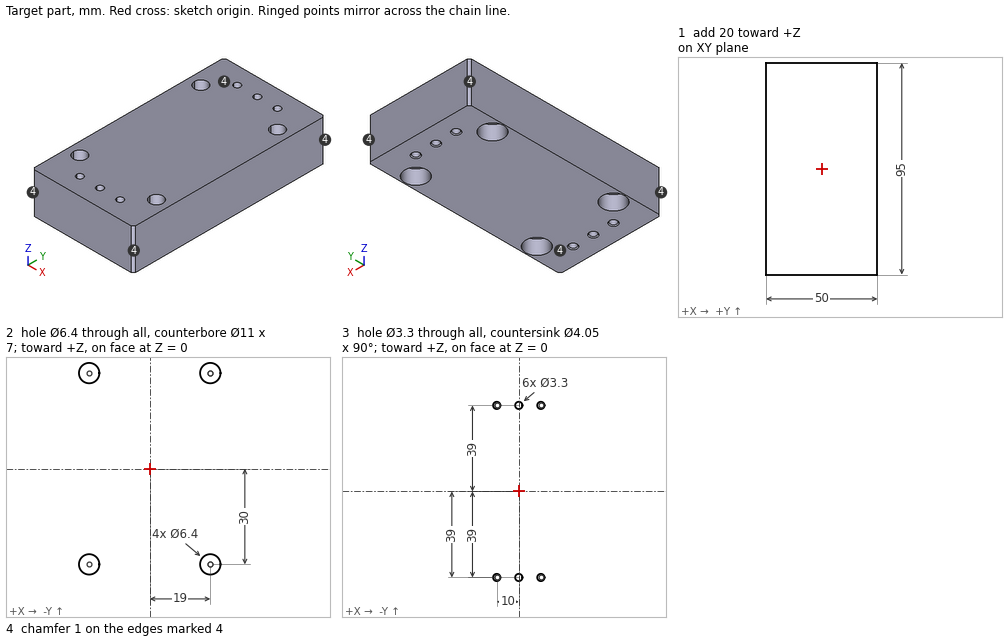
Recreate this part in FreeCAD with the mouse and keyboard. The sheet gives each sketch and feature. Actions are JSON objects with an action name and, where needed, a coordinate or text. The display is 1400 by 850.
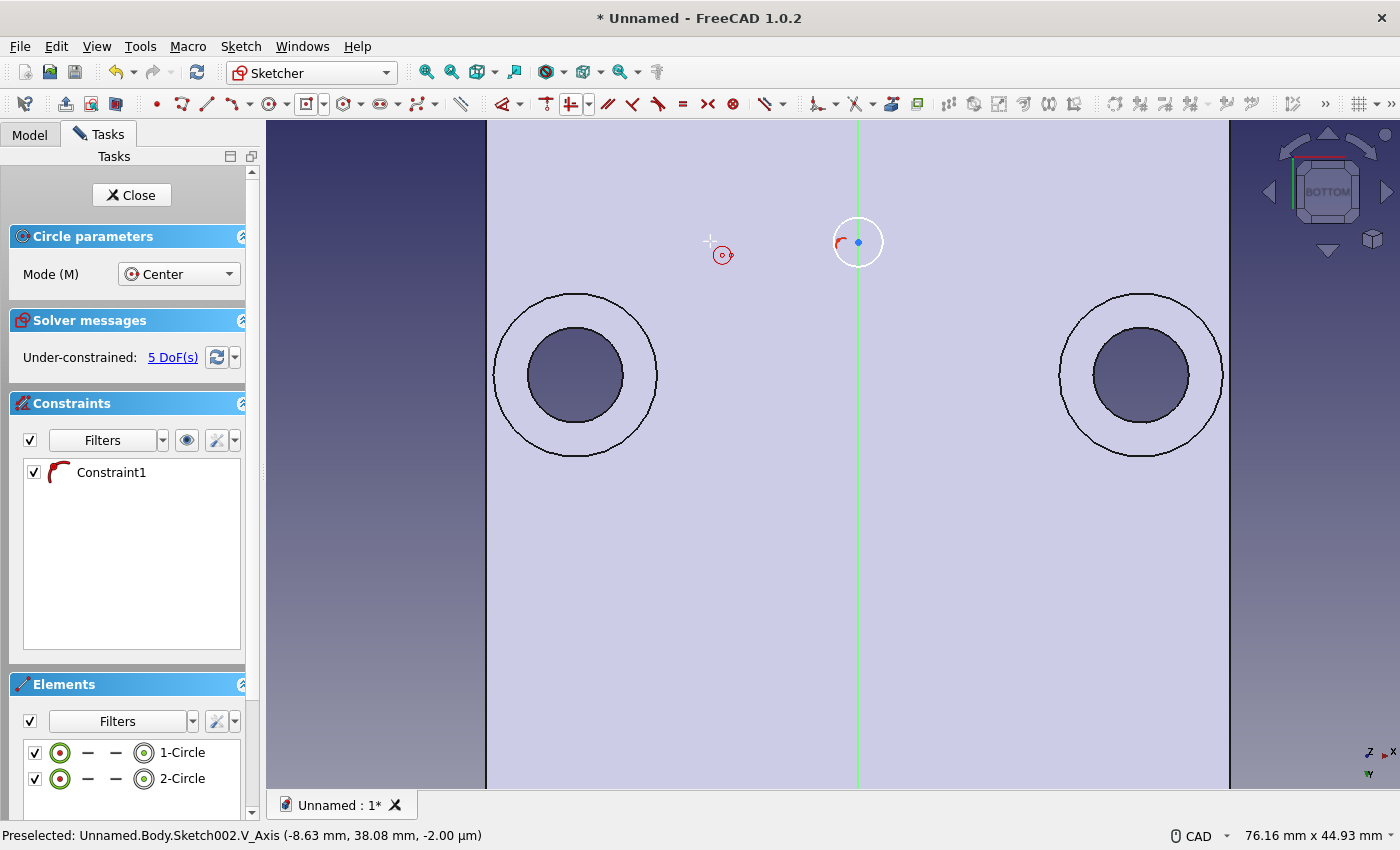
{"action": "left_click", "coordinate": [709, 241]}
{"action": "left_click", "coordinate": [727, 224]}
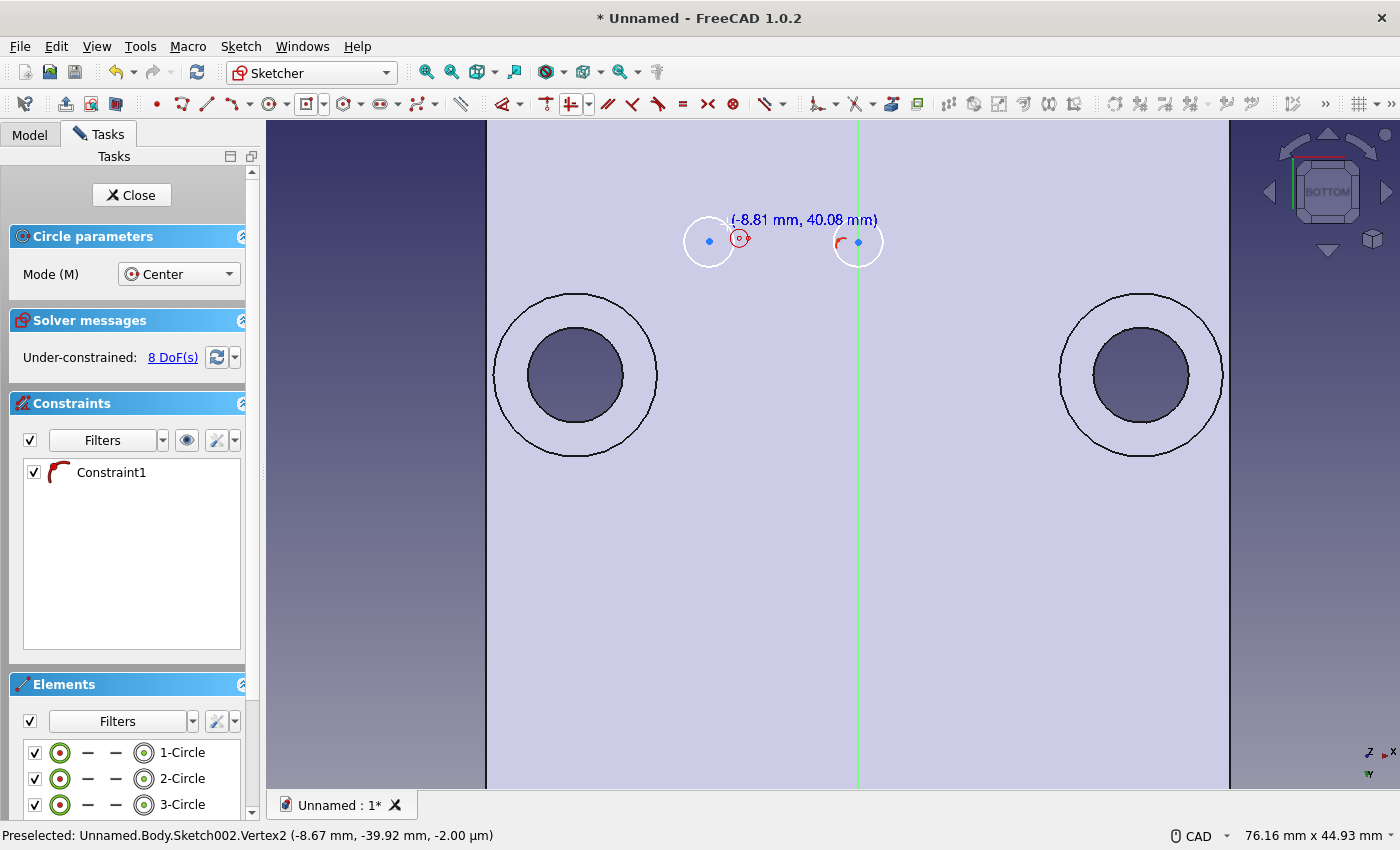
{"action": "left_click", "coordinate": [1007, 241]}
{"action": "left_click", "coordinate": [1024, 224]}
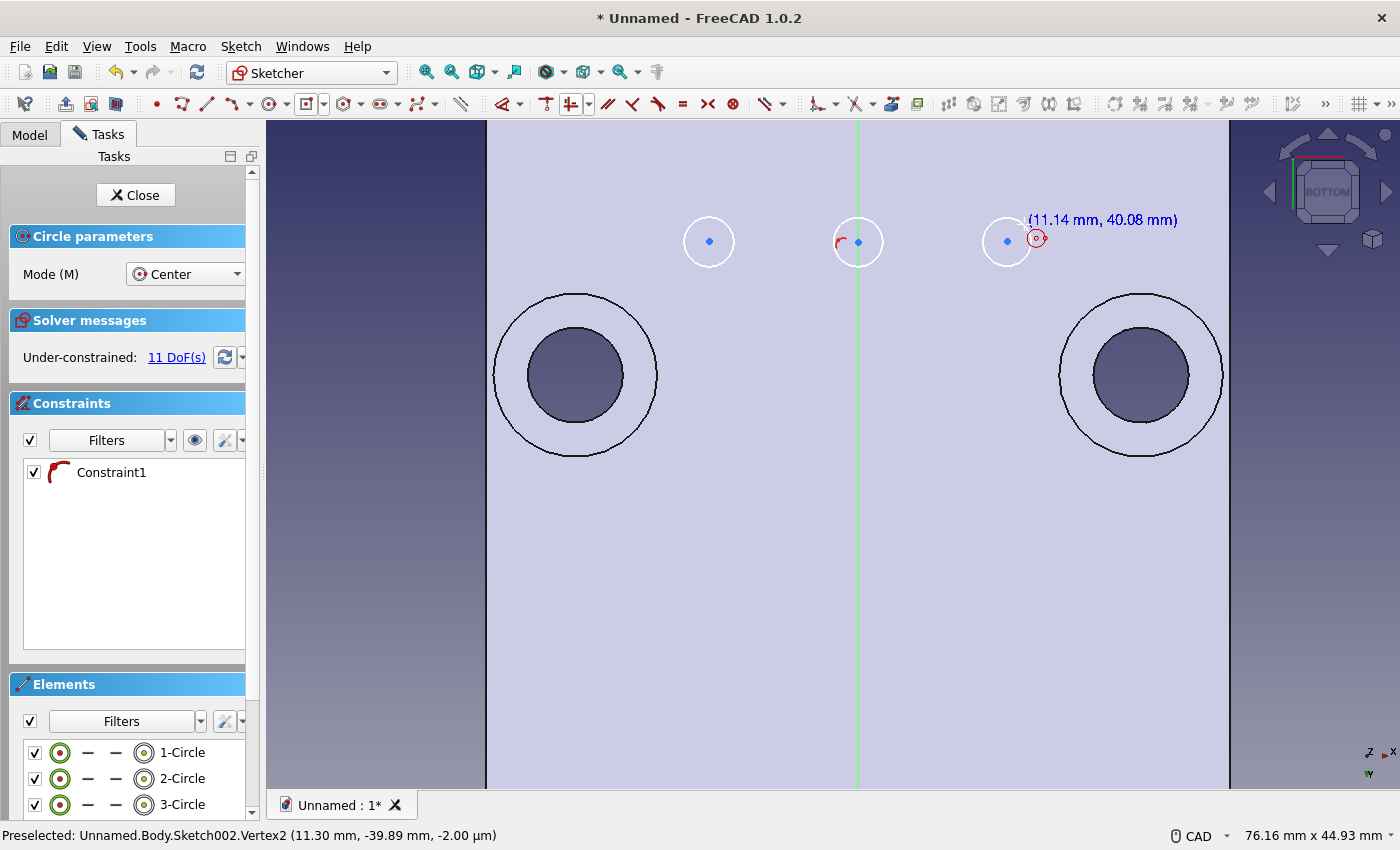
{"action": "scroll", "coordinate": [710, 241], "scroll_direction": "down", "scroll_amount": 5}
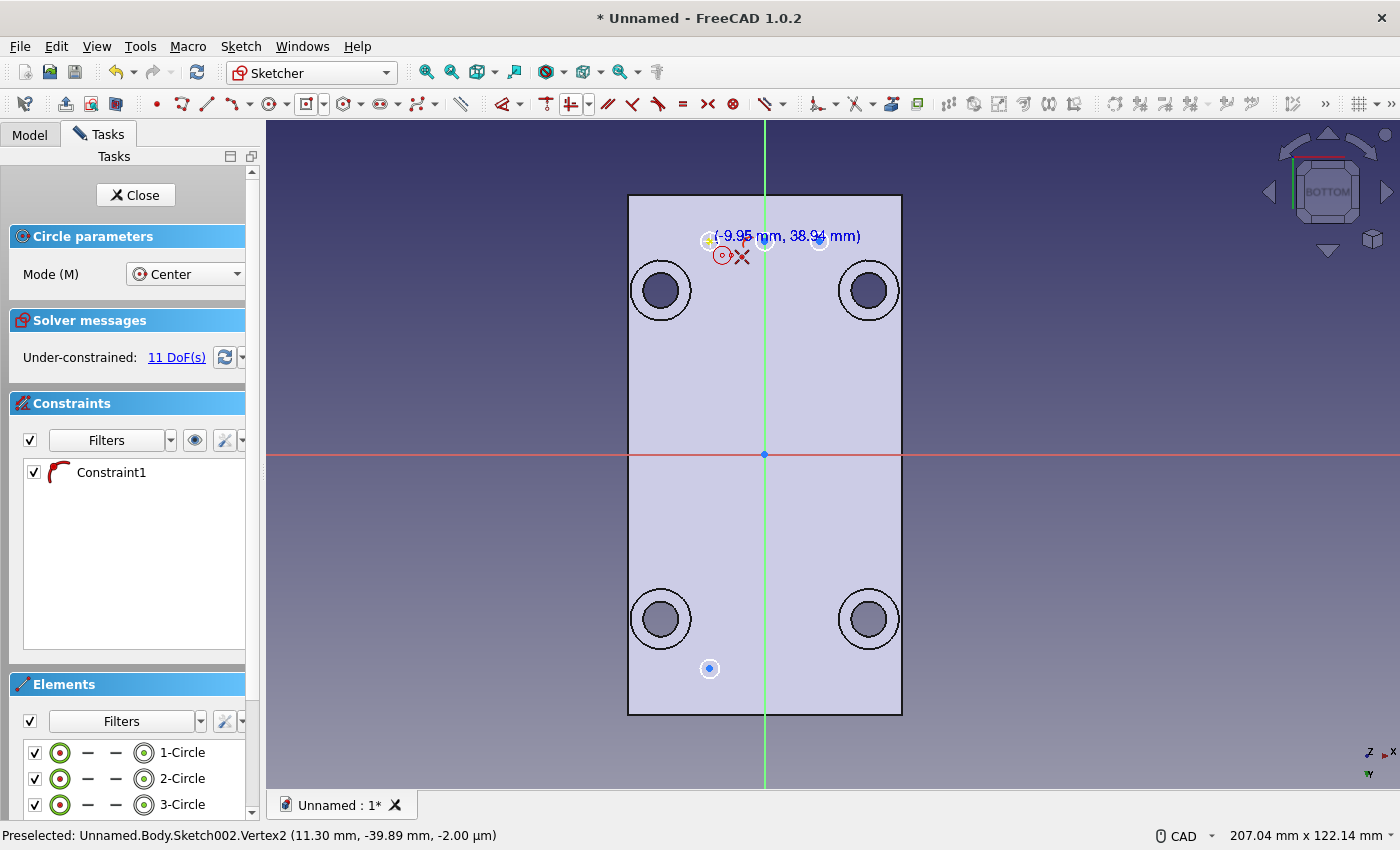
{"action": "scroll", "coordinate": [820, 668], "scroll_direction": "up", "scroll_amount": 5}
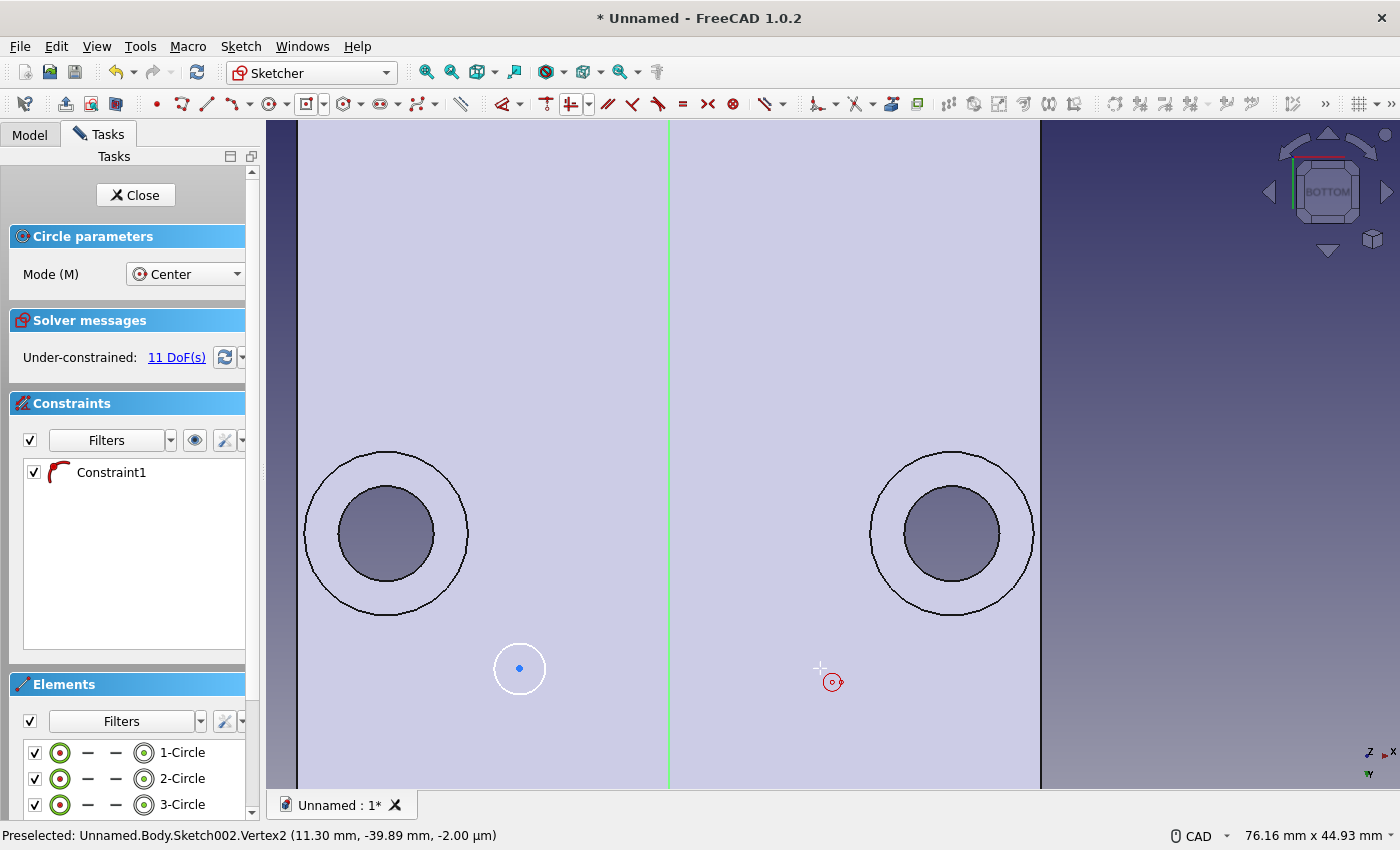
{"action": "left_click", "coordinate": [818, 668]}
{"action": "left_click", "coordinate": [835, 650]}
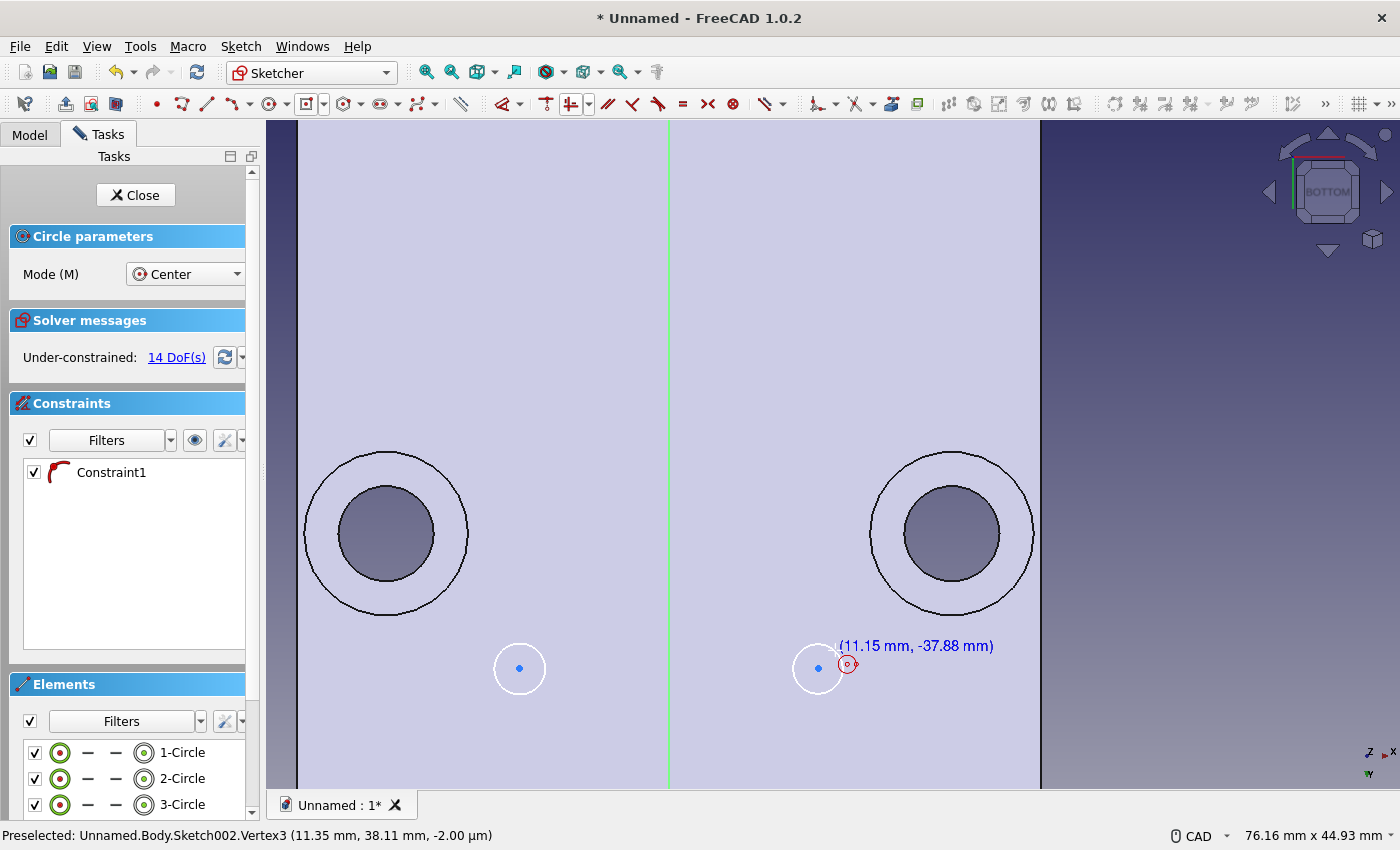
{"action": "left_click", "coordinate": [669, 668]}
{"action": "left_click", "coordinate": [686, 650]}
{"action": "key", "text": "Escape"}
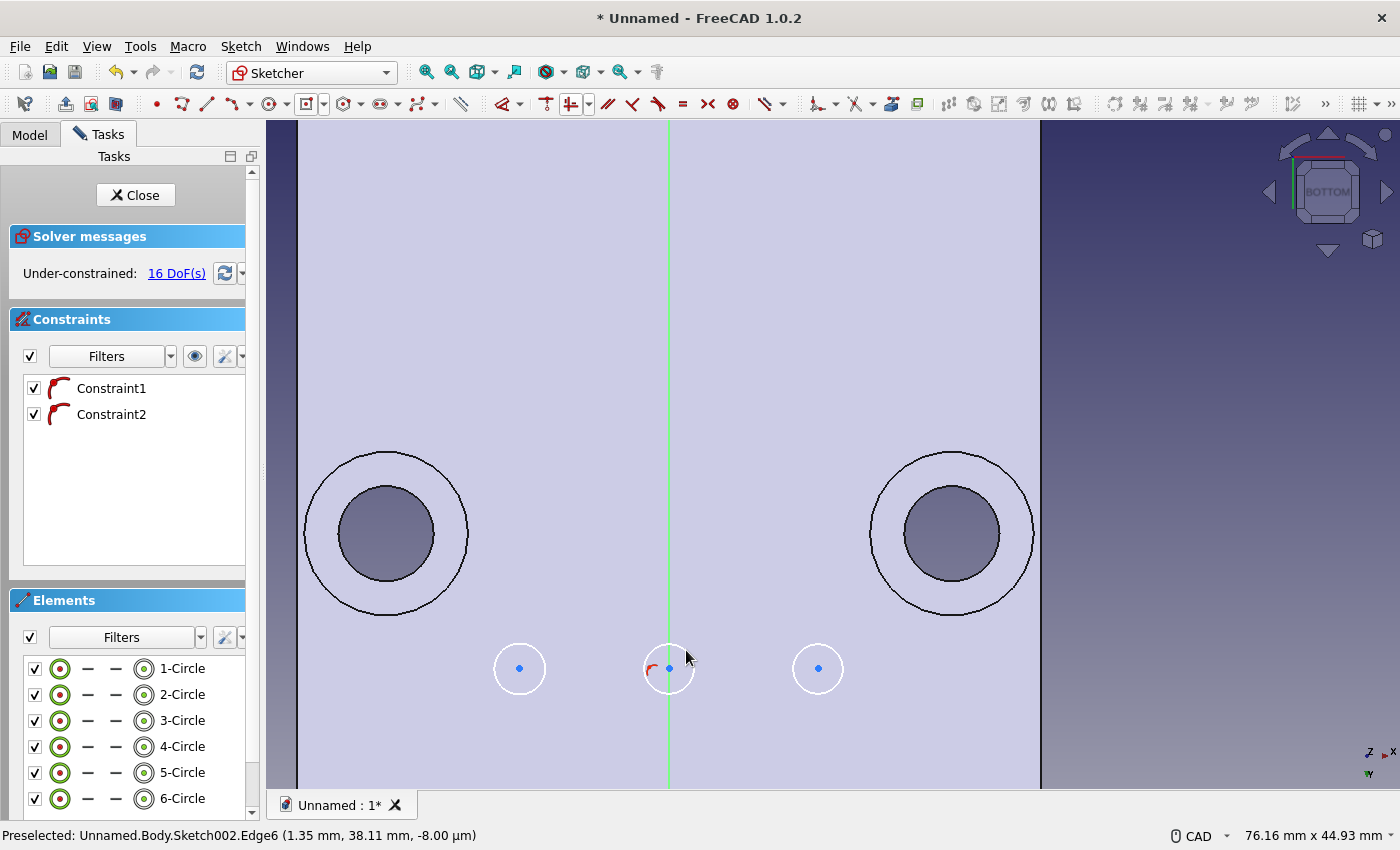
{"action": "scroll", "coordinate": [820, 668], "scroll_direction": "down", "scroll_amount": 5}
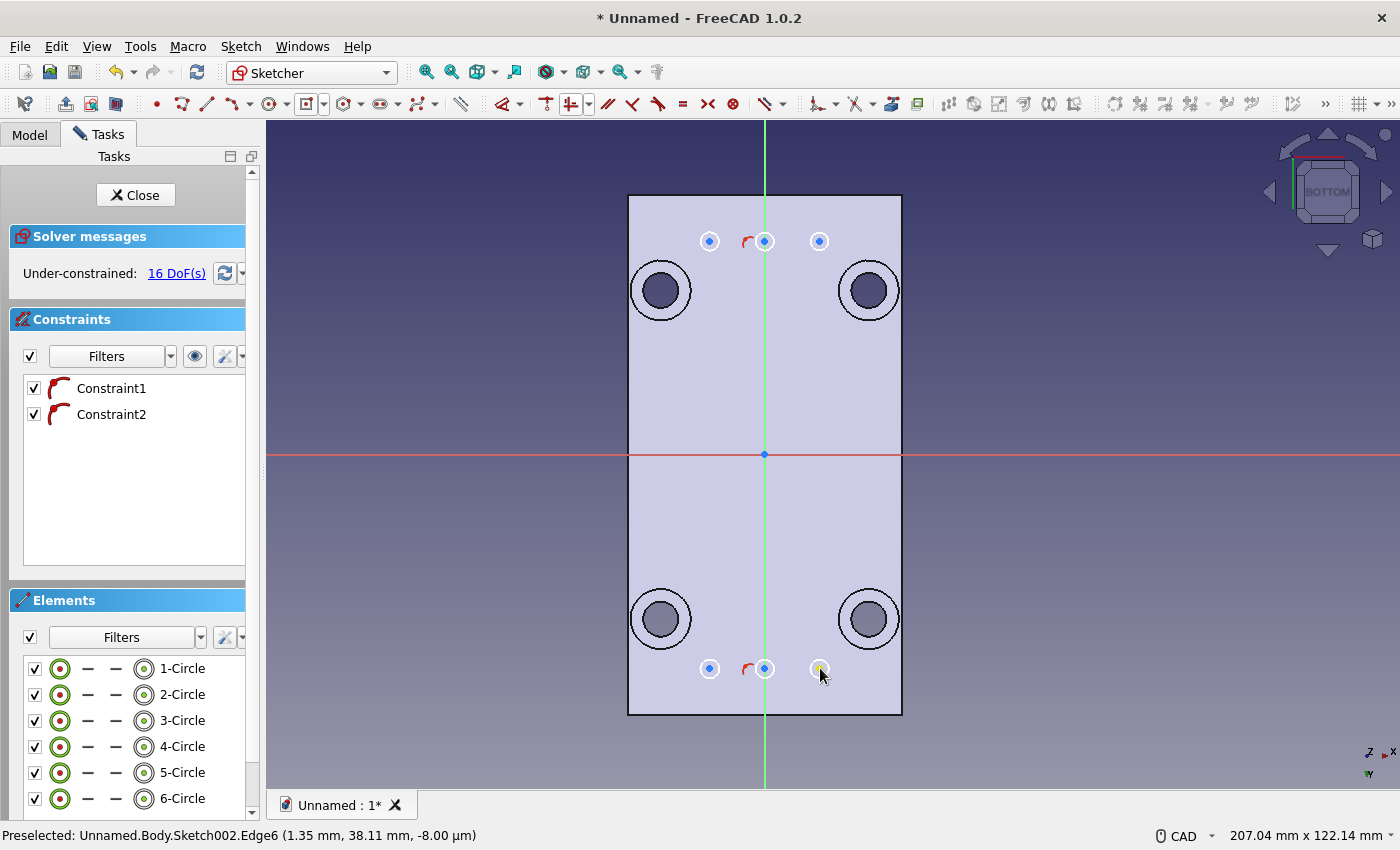
{"action": "scroll", "coordinate": [771, 235], "scroll_direction": "up", "scroll_amount": 4}